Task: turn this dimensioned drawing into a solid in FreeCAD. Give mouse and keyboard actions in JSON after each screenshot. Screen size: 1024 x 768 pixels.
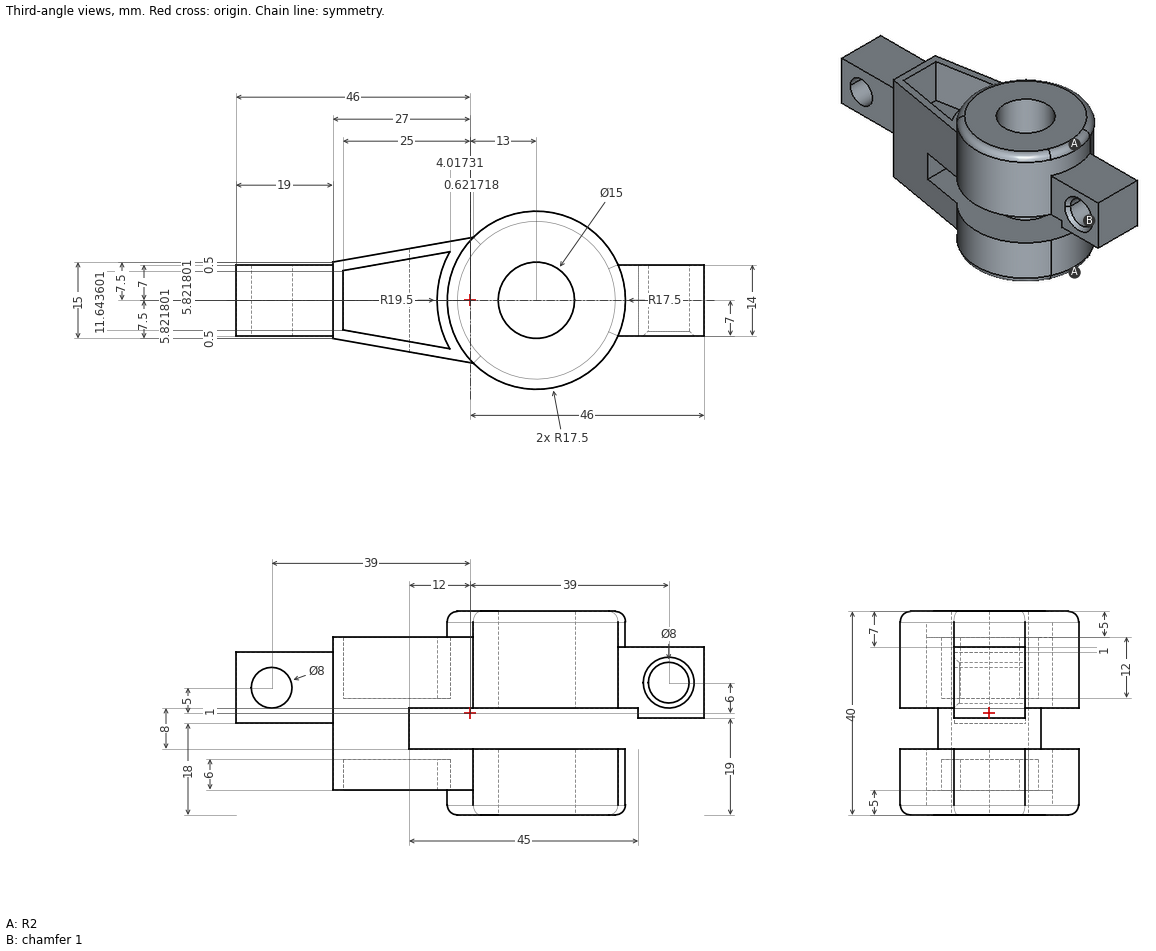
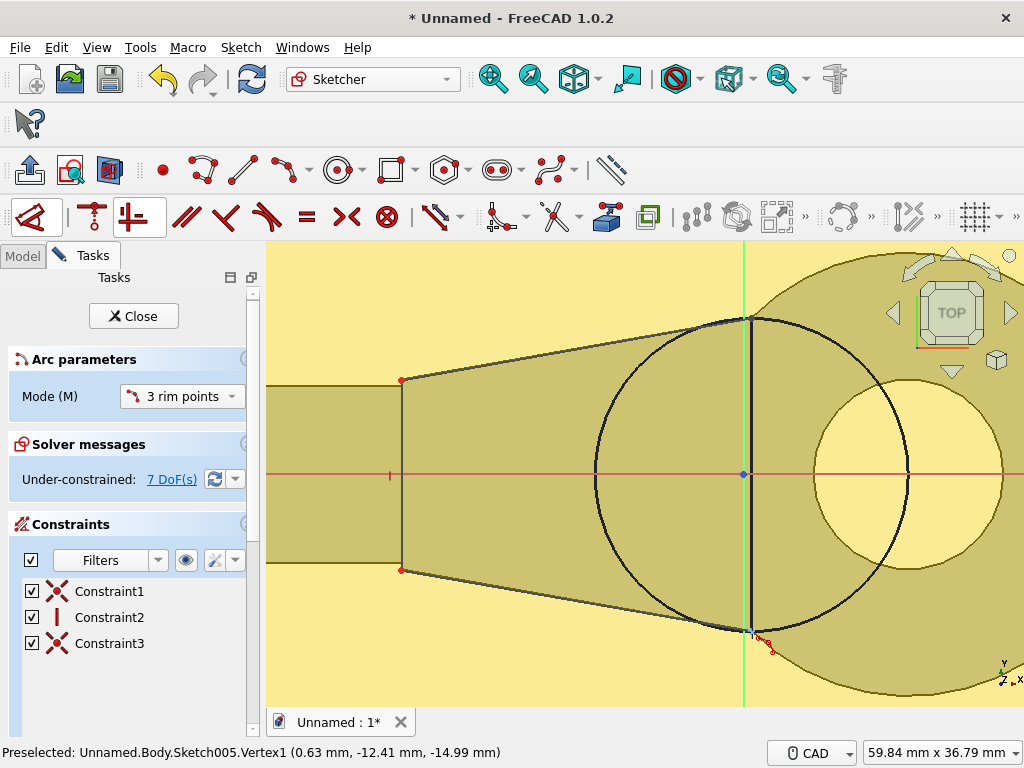
{"action": "left_click", "coordinate": [689, 440]}
{"action": "key", "text": "Escape"}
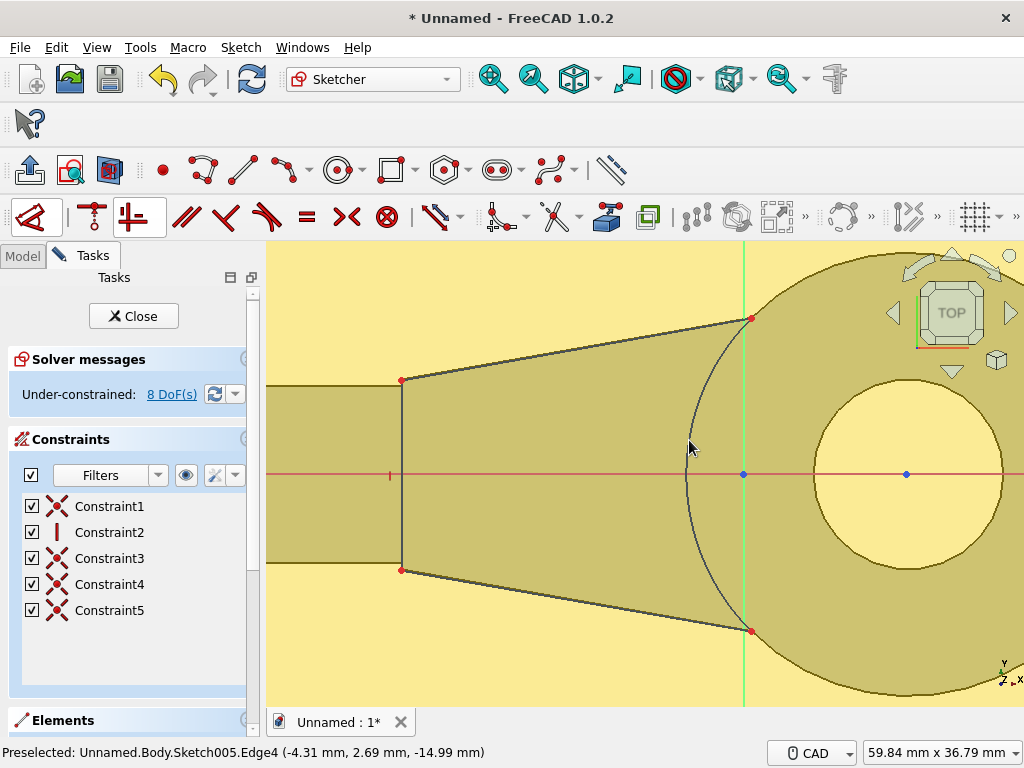
{"action": "scroll", "coordinate": [294, 472], "scroll_direction": "down", "scroll_amount": 1}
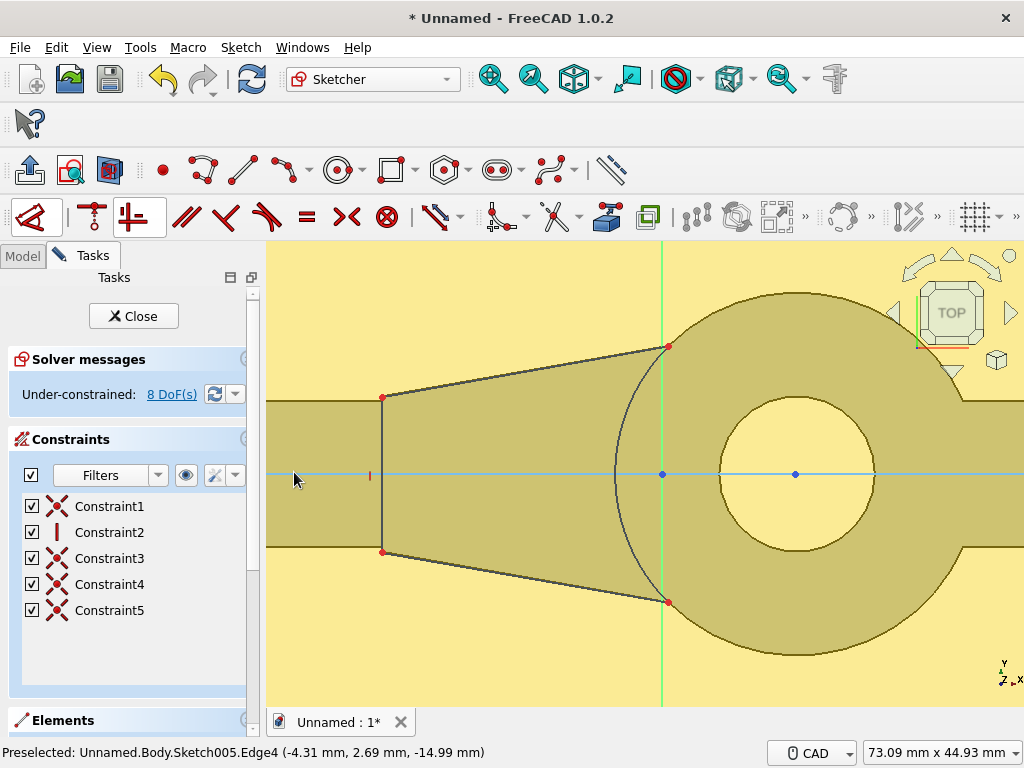
{"action": "left_click", "coordinate": [796, 475]}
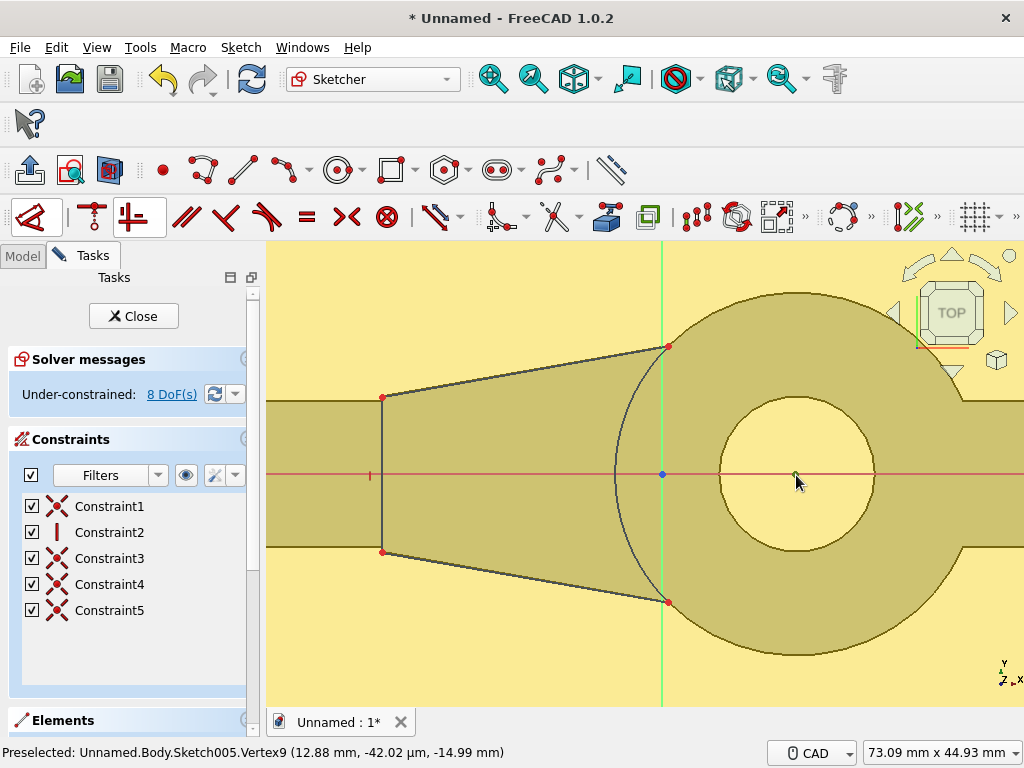
{"action": "left_click", "coordinate": [334, 474]}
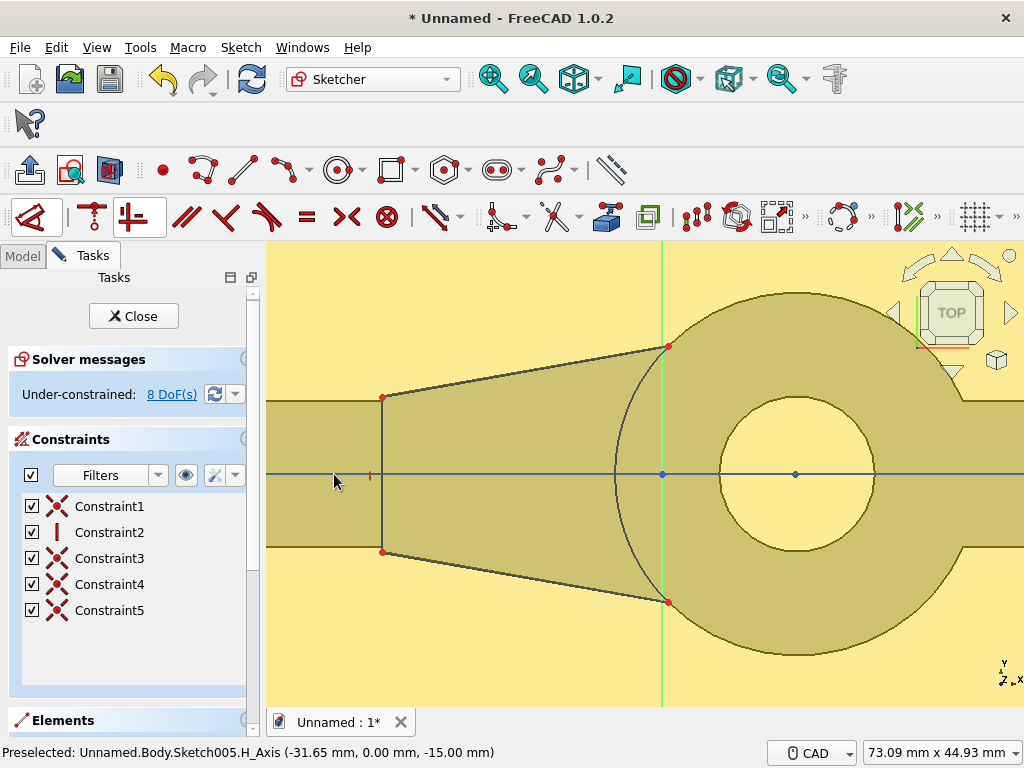
{"action": "left_click", "coordinate": [92, 218]}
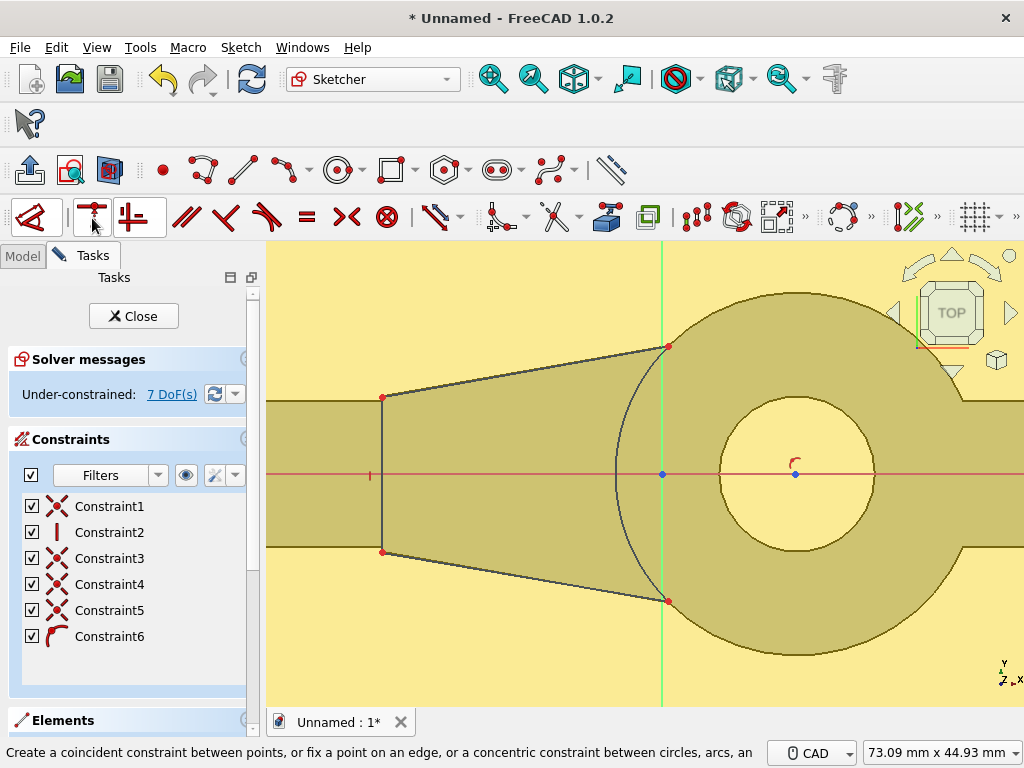
{"action": "left_click", "coordinate": [624, 418]}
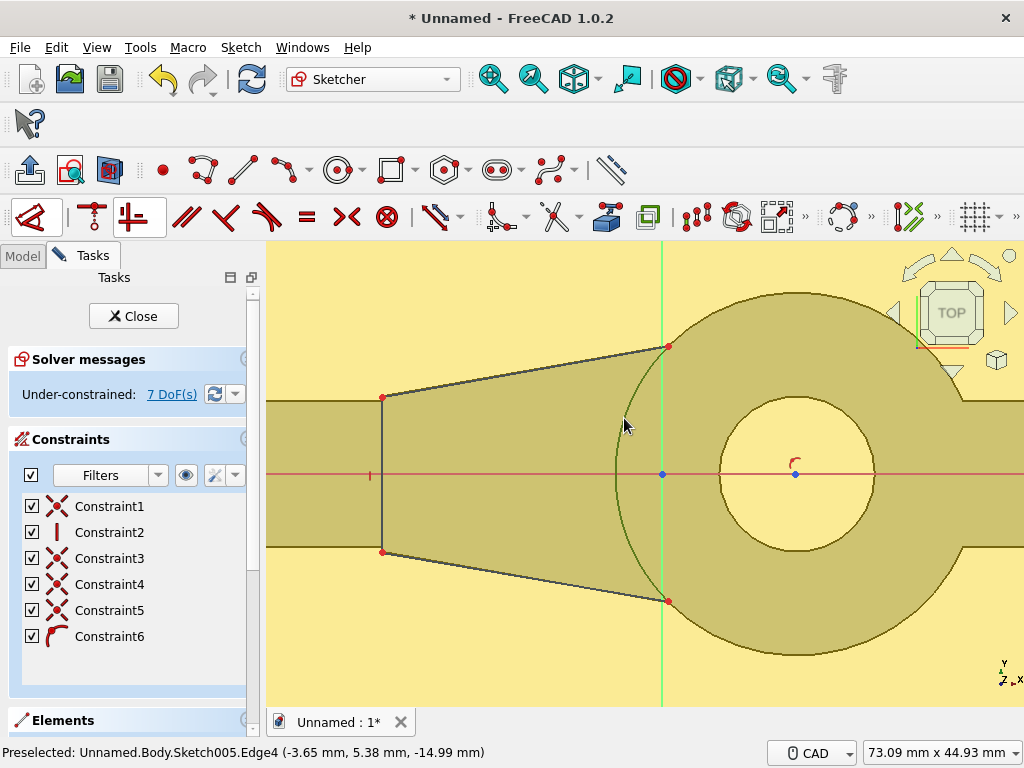
{"action": "left_click", "coordinate": [56, 218]}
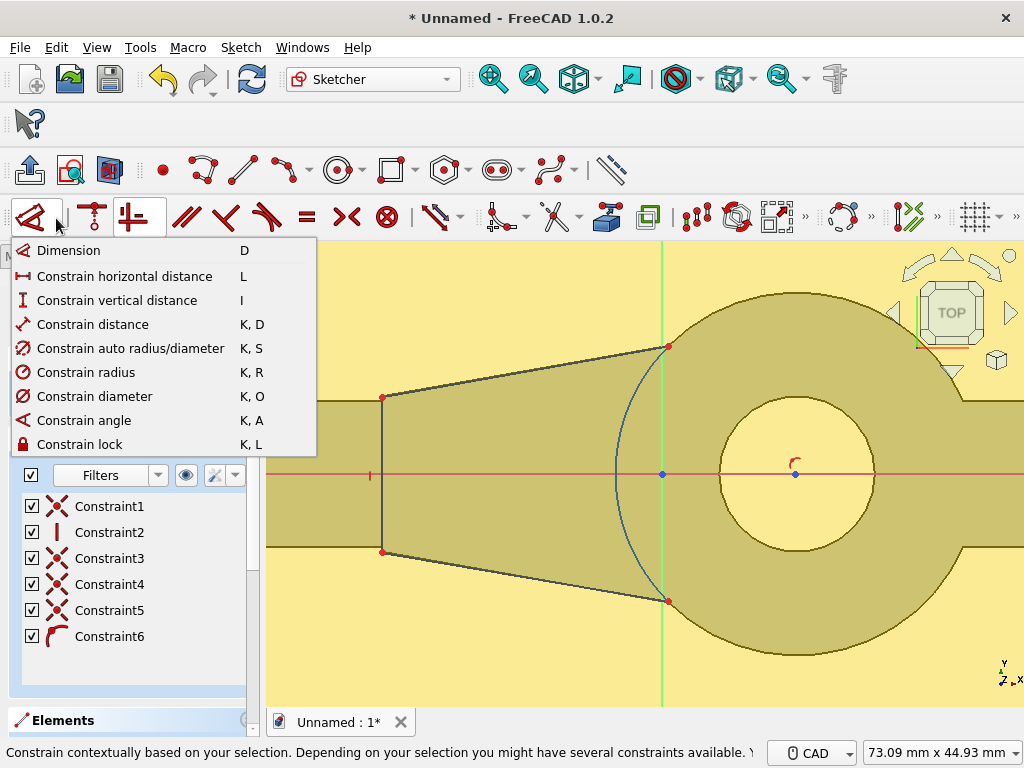
{"action": "left_click", "coordinate": [164, 372]}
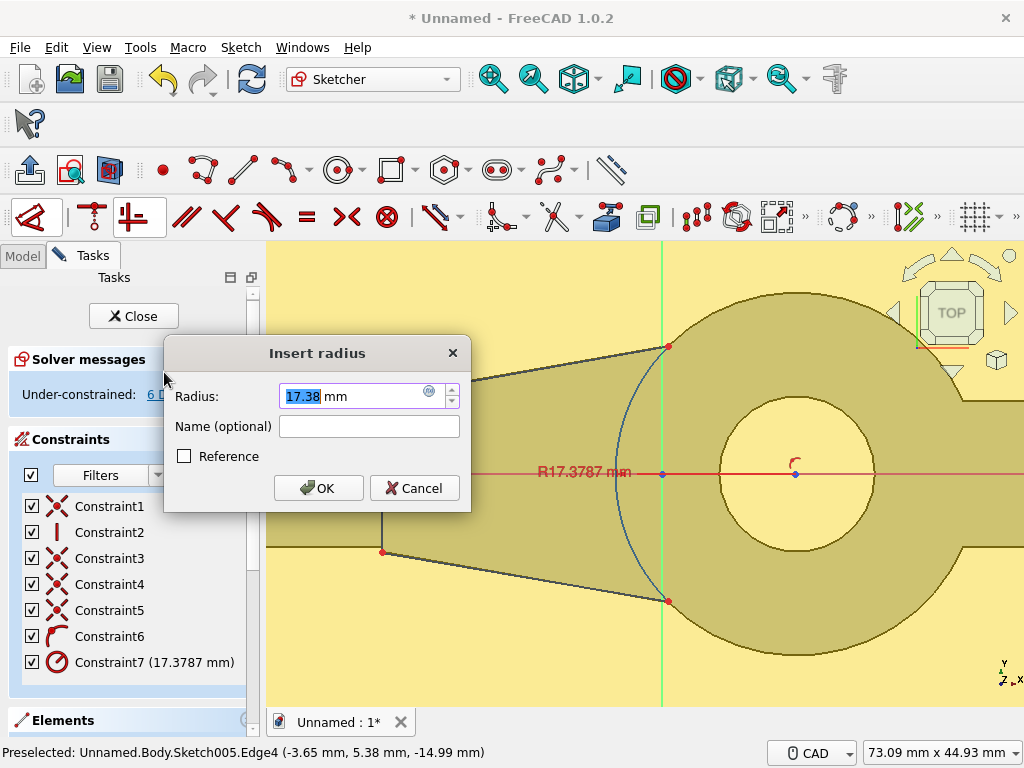
{"action": "type", "text": "17.5"}
{"action": "key", "text": "Return"}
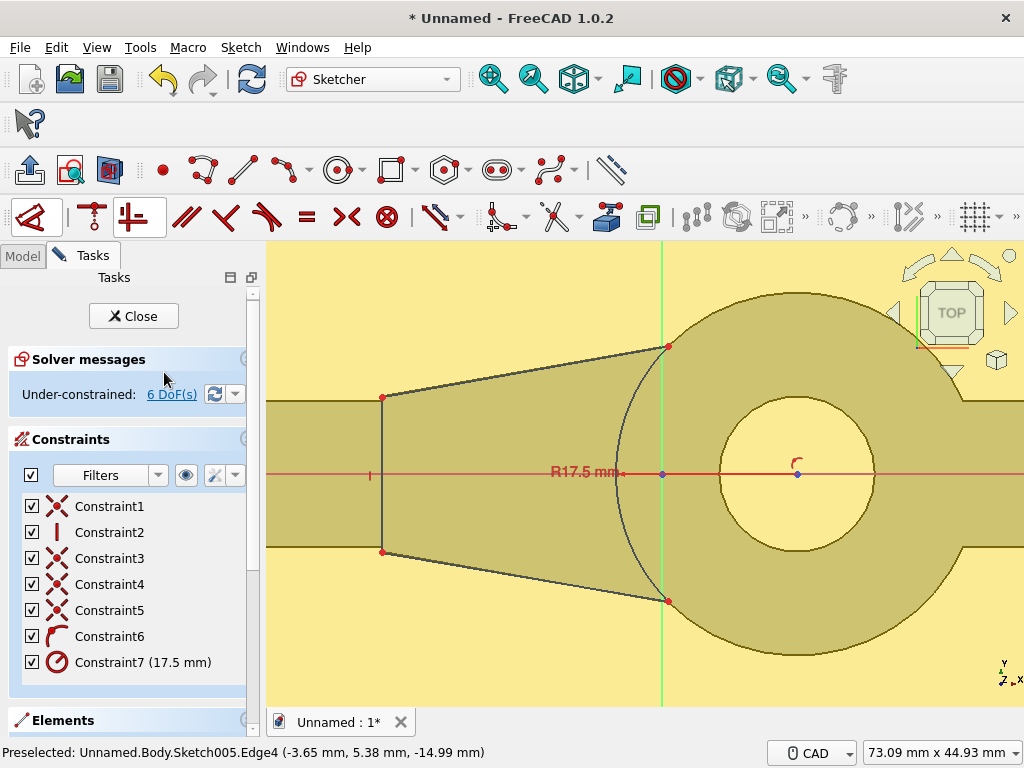
{"action": "left_click", "coordinate": [382, 506]}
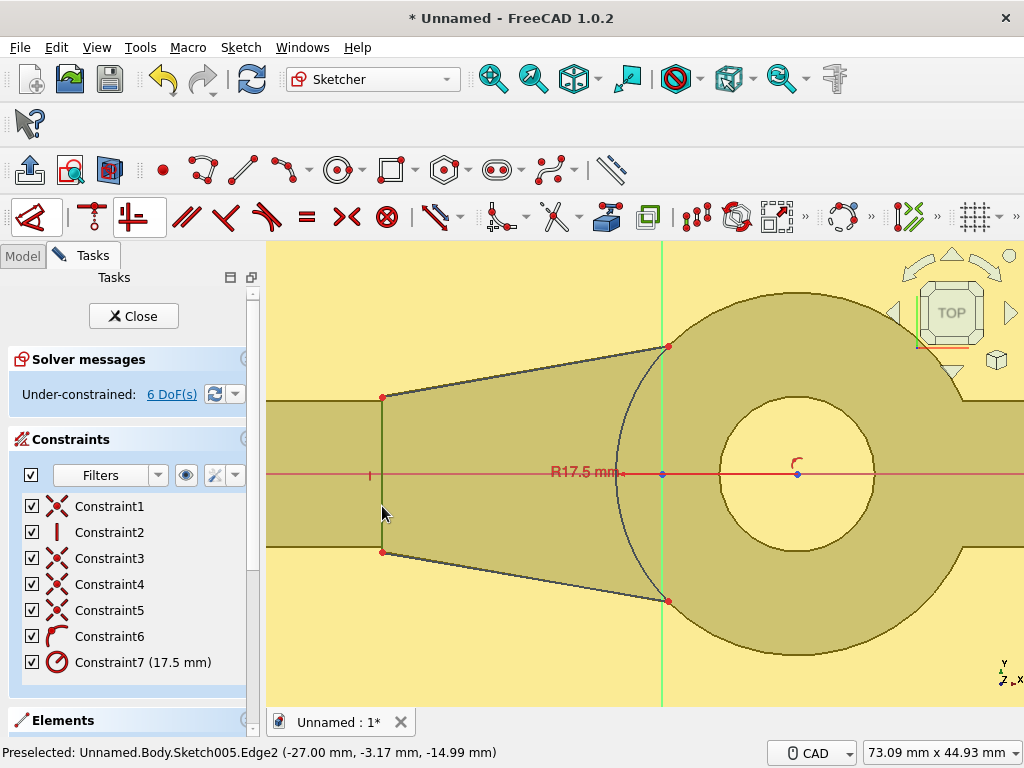
{"action": "left_click", "coordinate": [56, 218]}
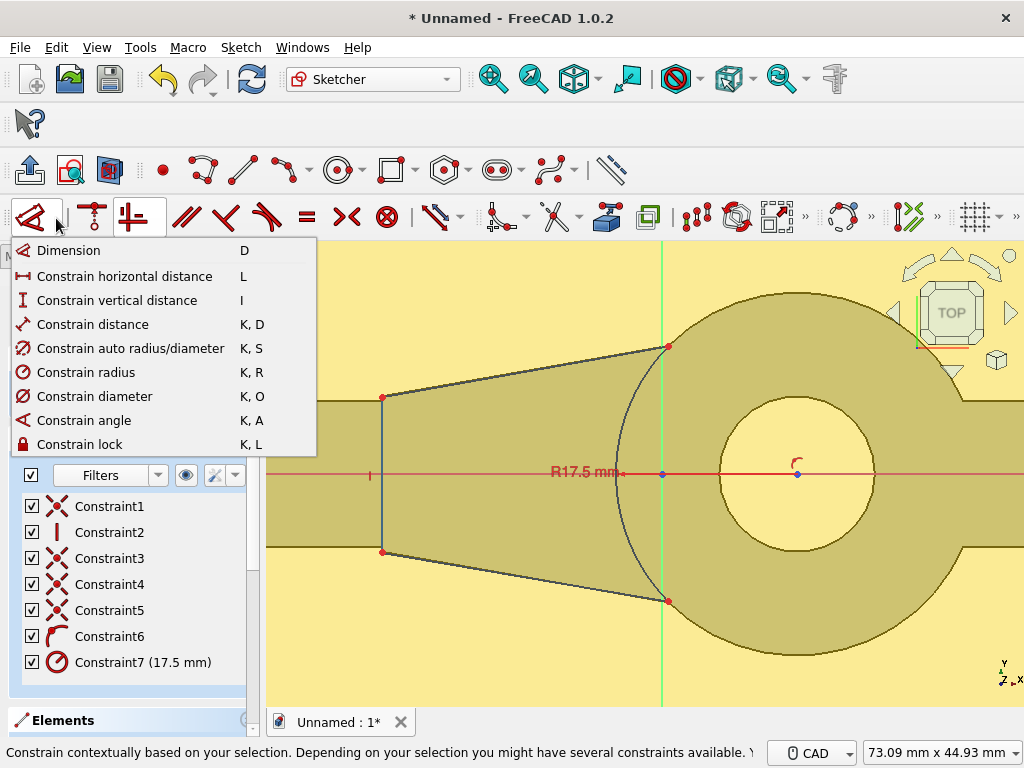
{"action": "left_click", "coordinate": [164, 300]}